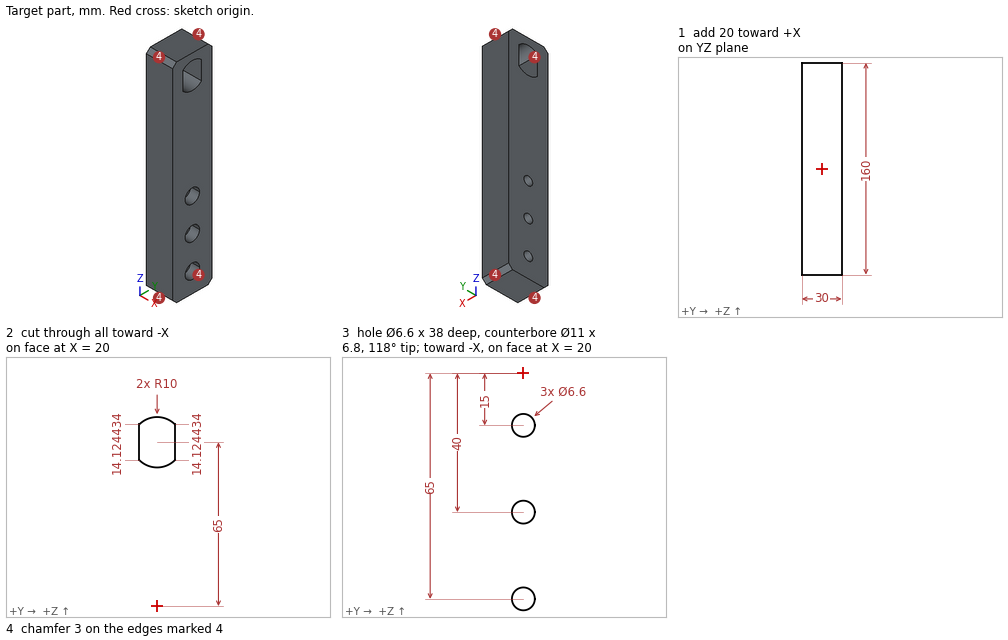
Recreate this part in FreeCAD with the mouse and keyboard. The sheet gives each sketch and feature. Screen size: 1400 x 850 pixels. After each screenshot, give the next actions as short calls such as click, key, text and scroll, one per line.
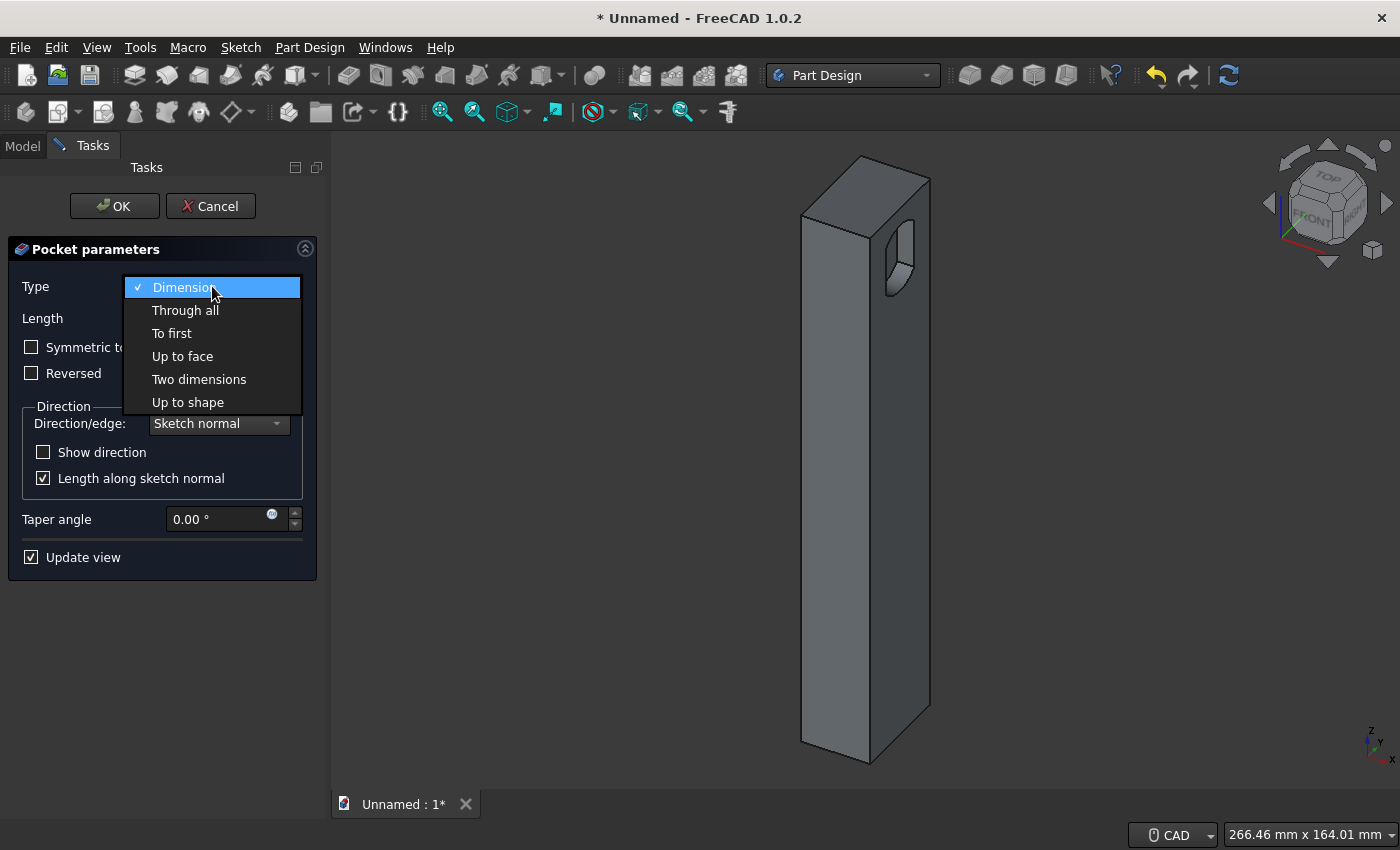
click(212, 310)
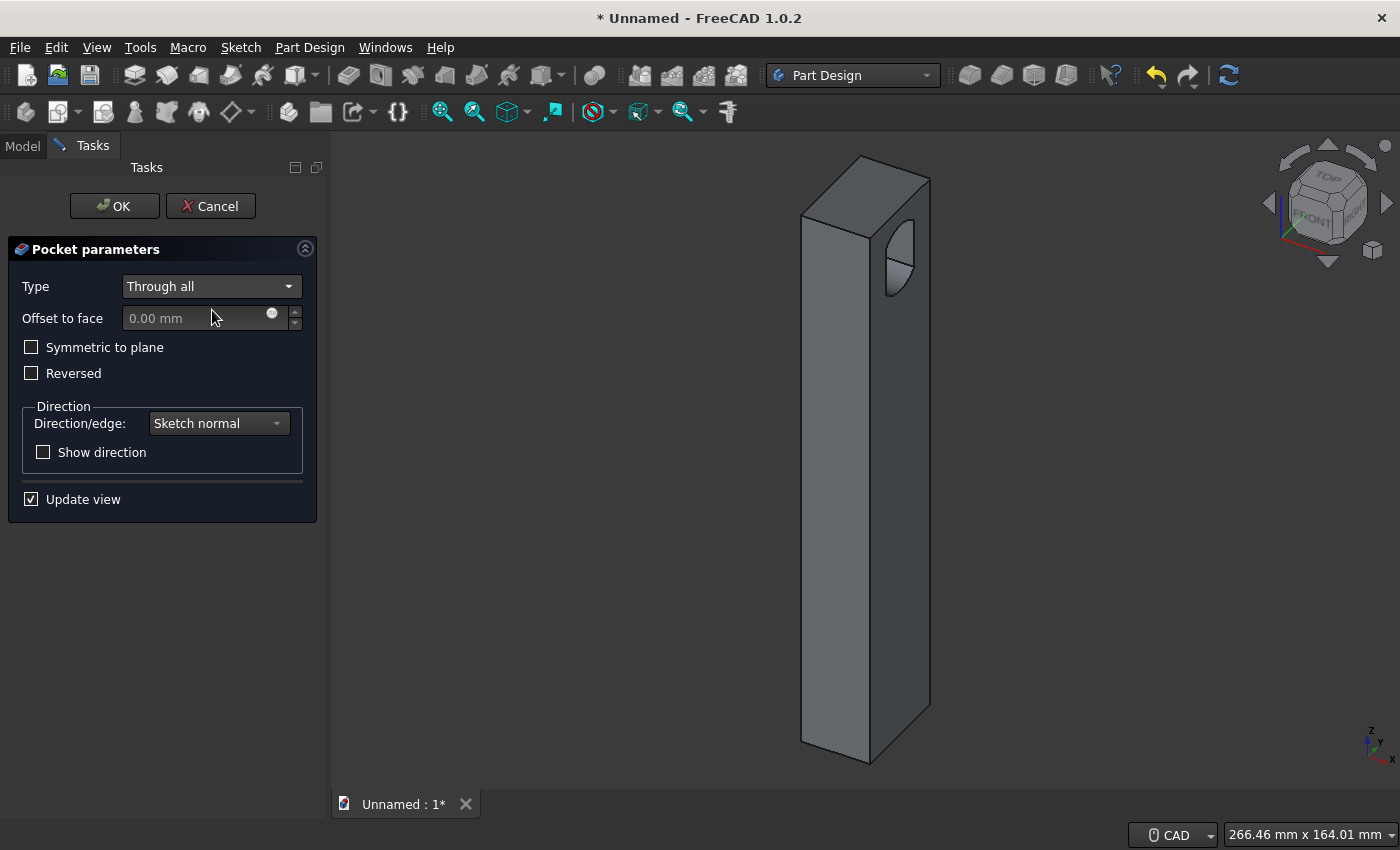
click(115, 206)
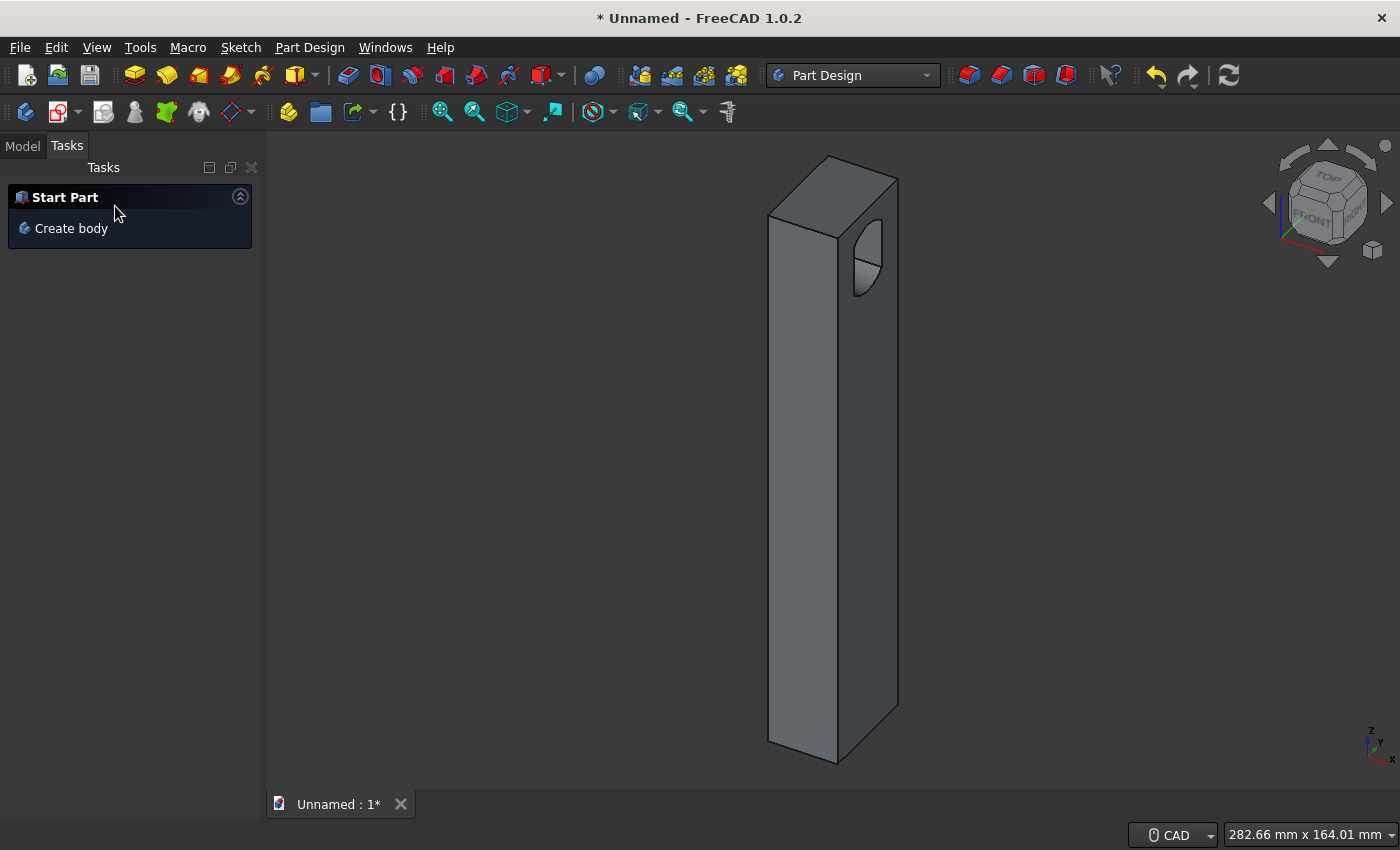
click(868, 621)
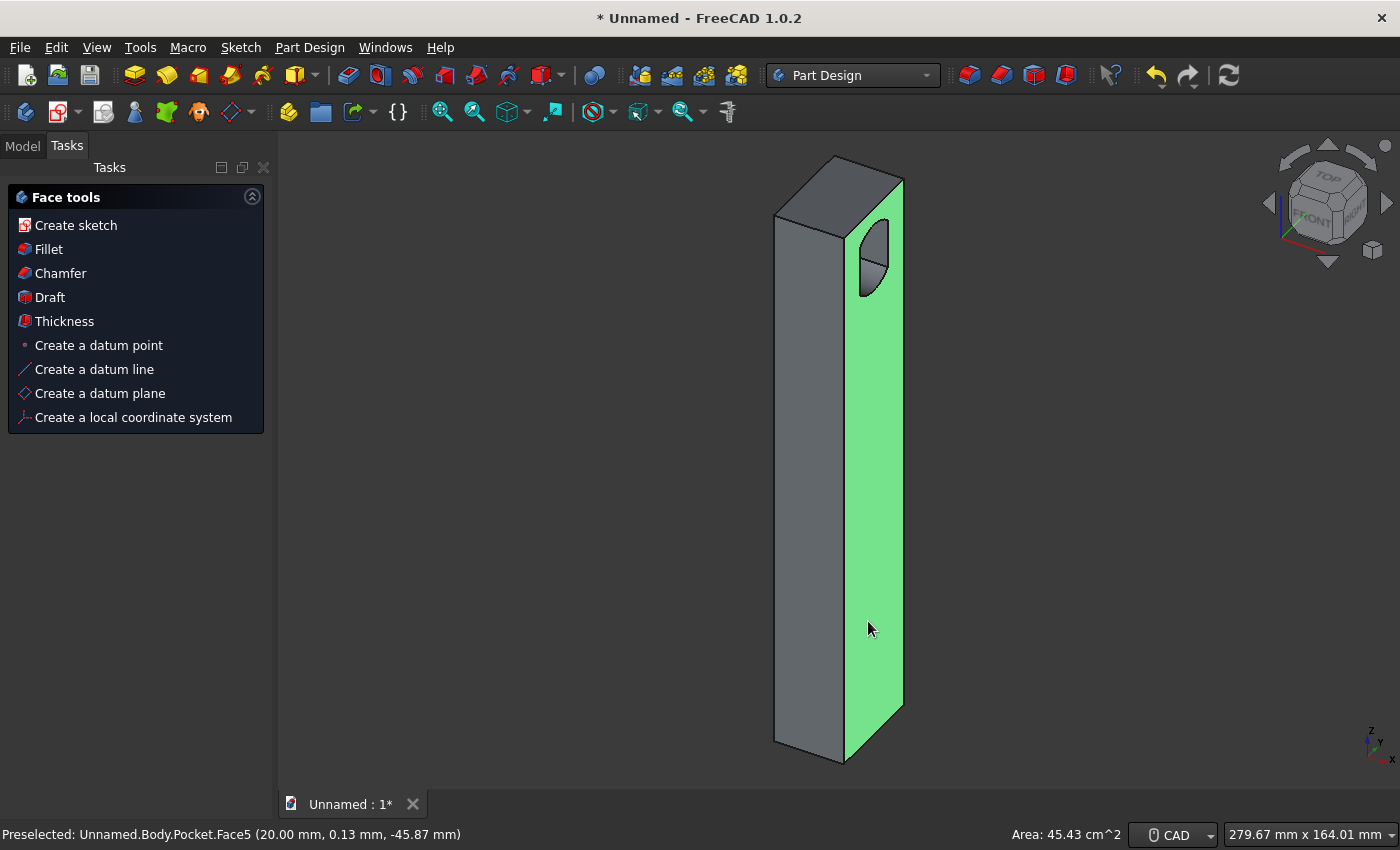
click(58, 112)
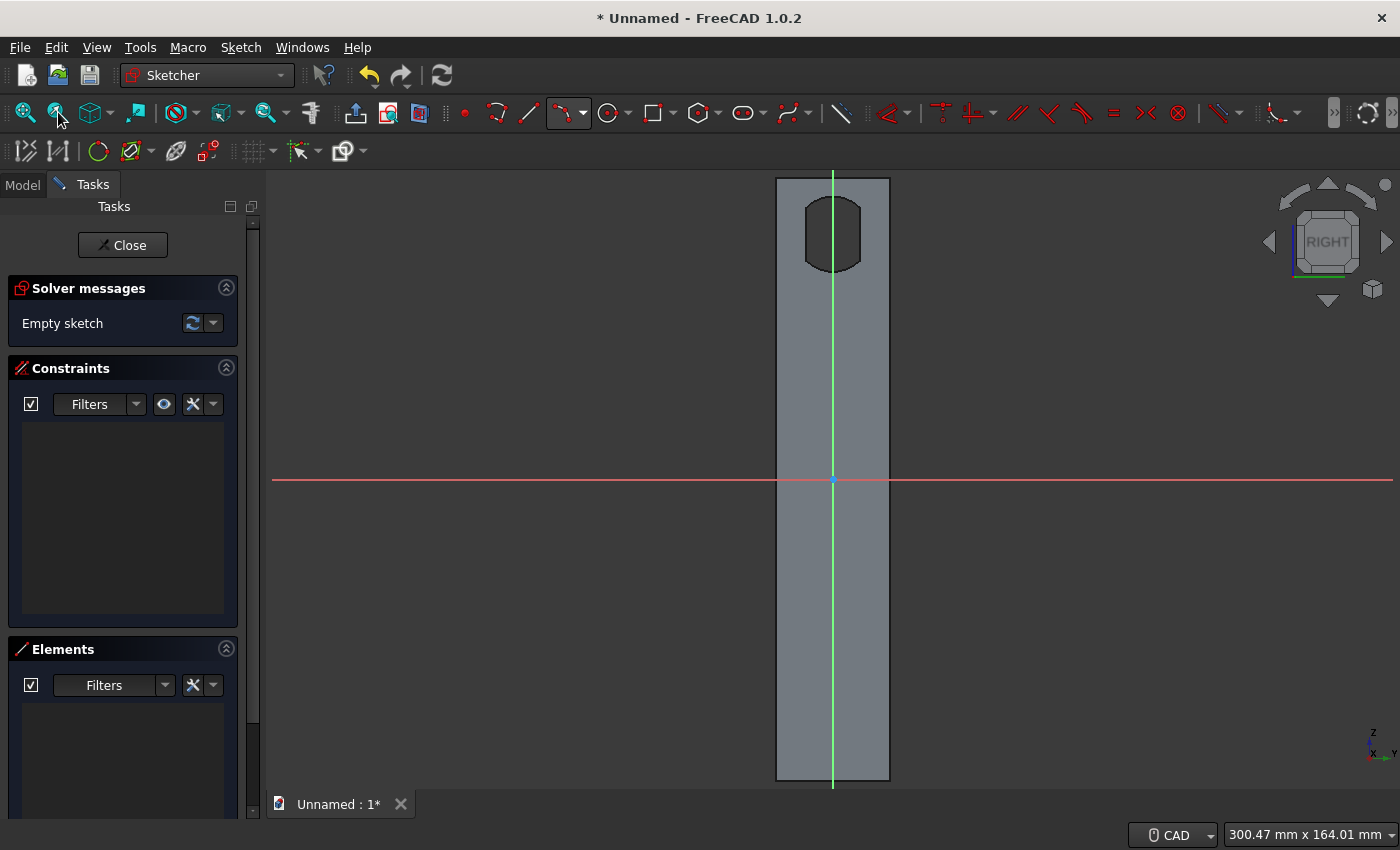
scroll(972, 761, up, 2)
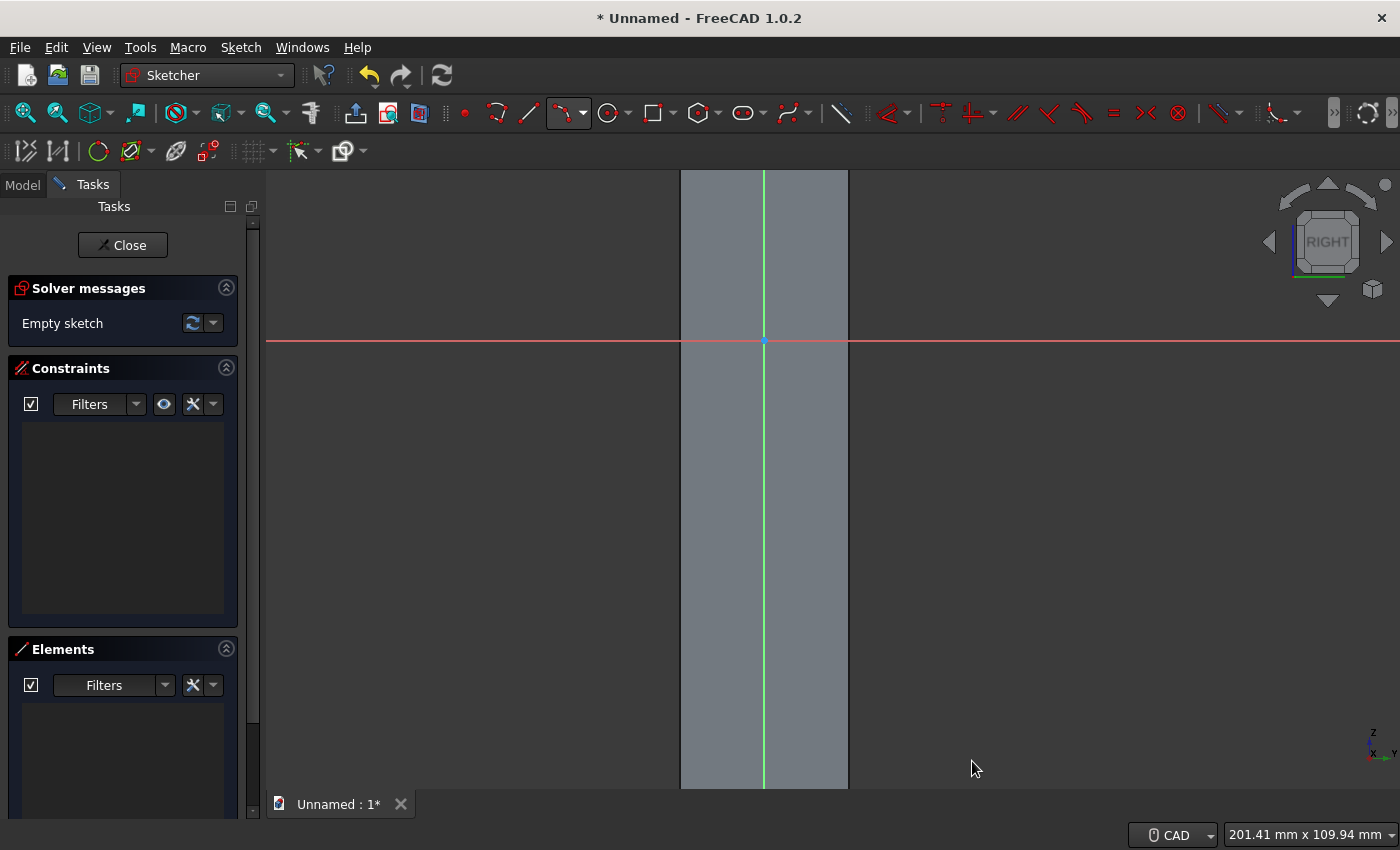
click(608, 114)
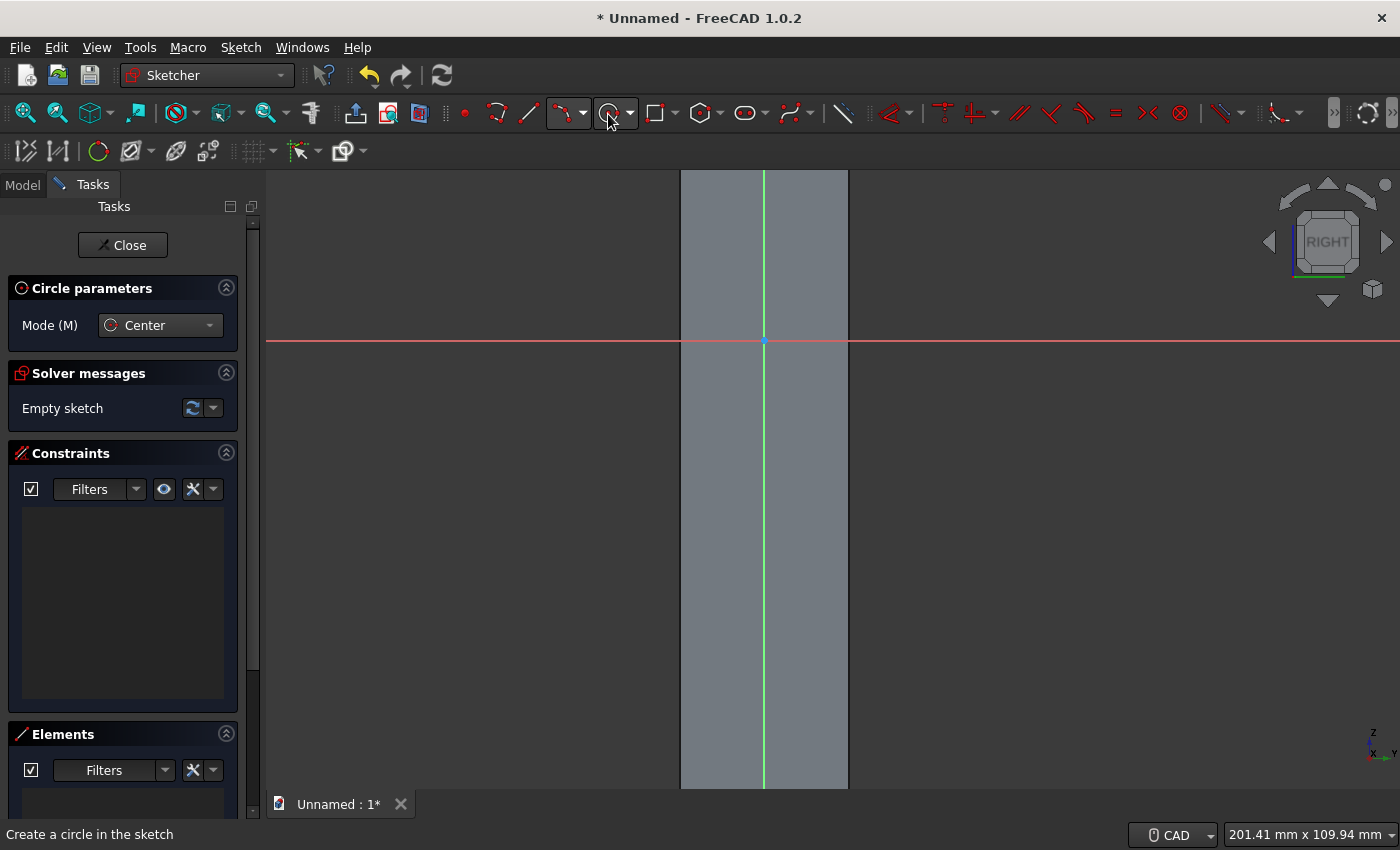
click(764, 425)
move(782, 419)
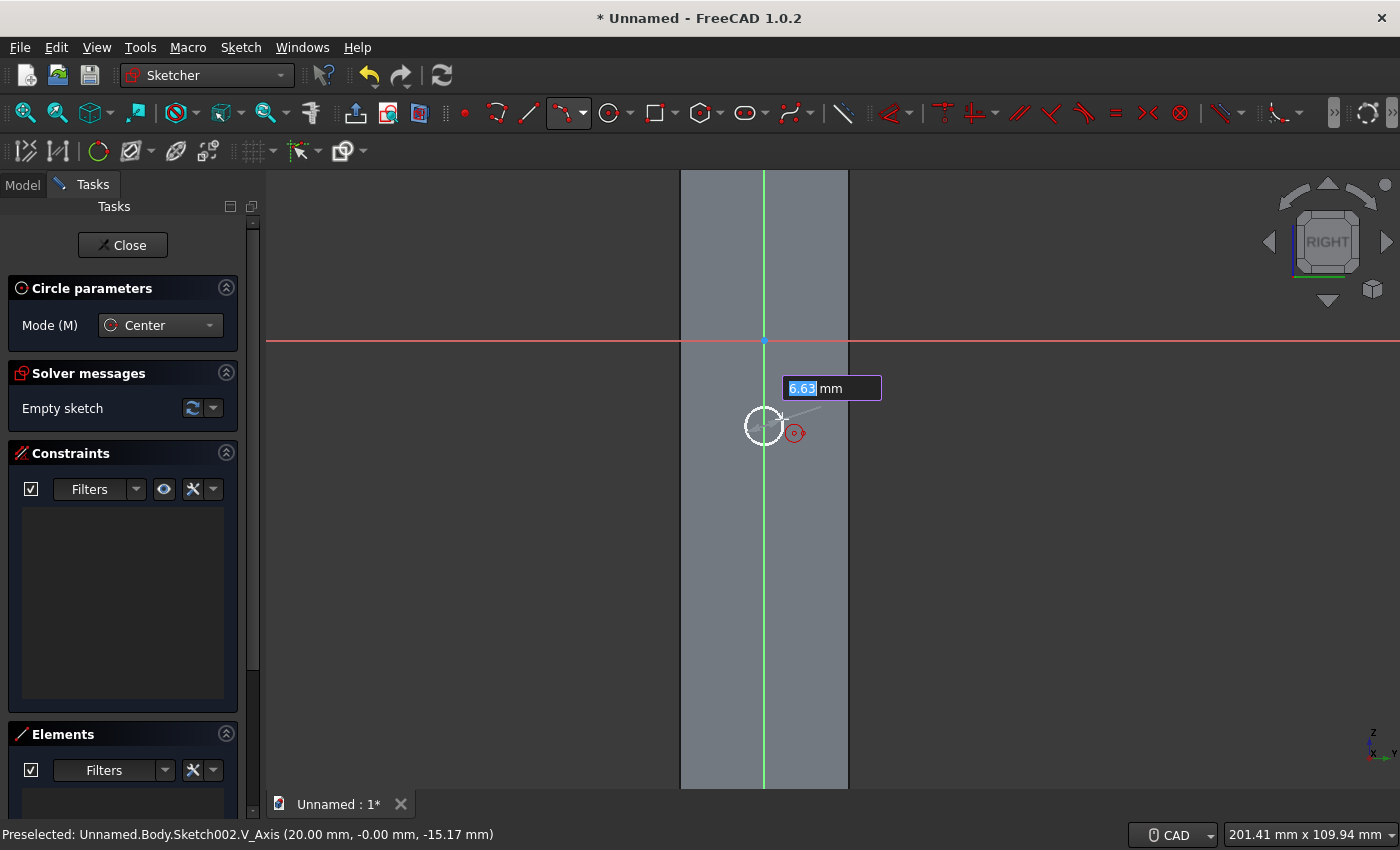
text(6.6)
key(Return)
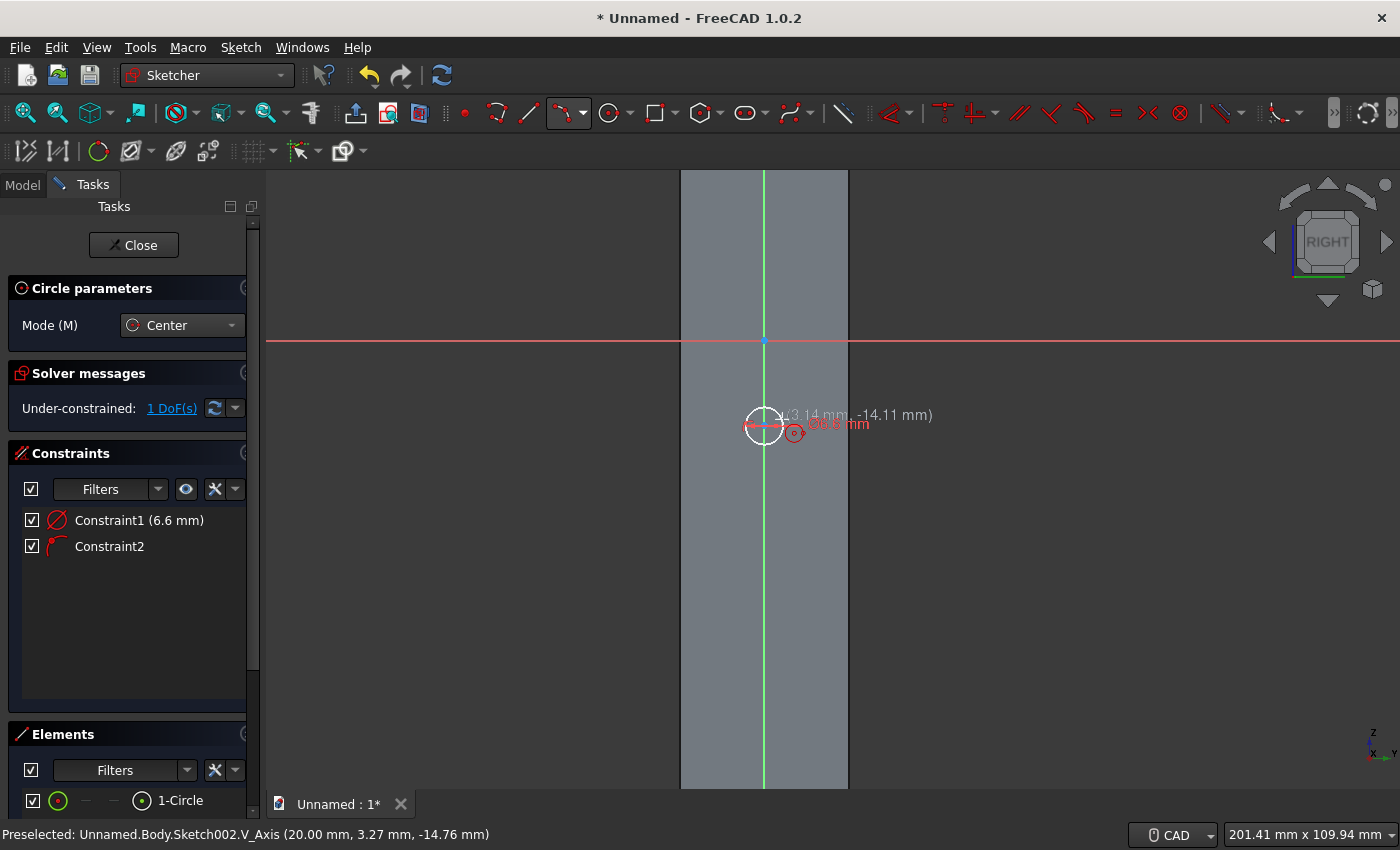
click(764, 566)
move(782, 559)